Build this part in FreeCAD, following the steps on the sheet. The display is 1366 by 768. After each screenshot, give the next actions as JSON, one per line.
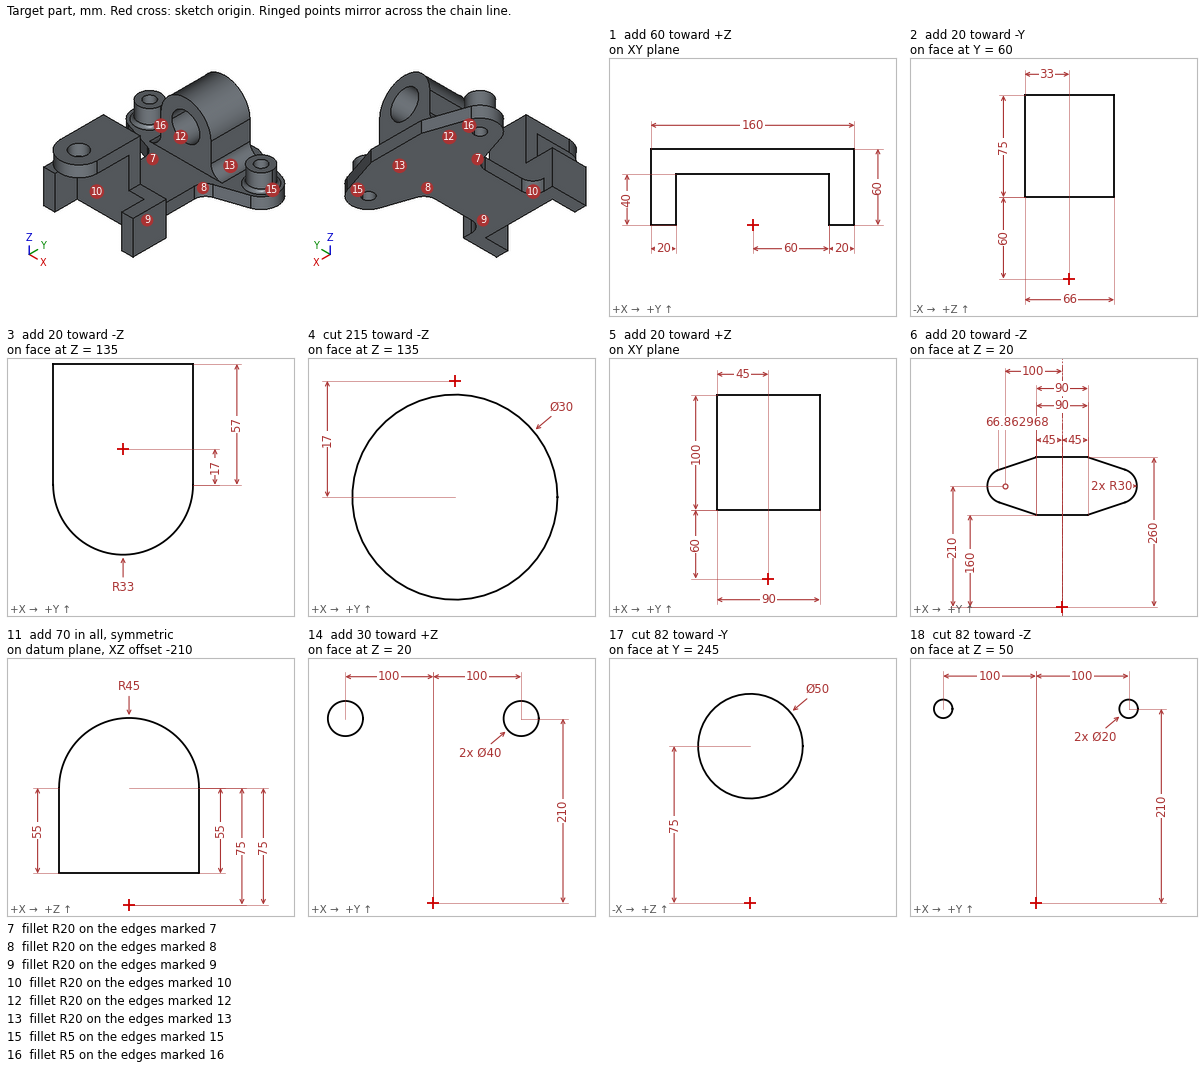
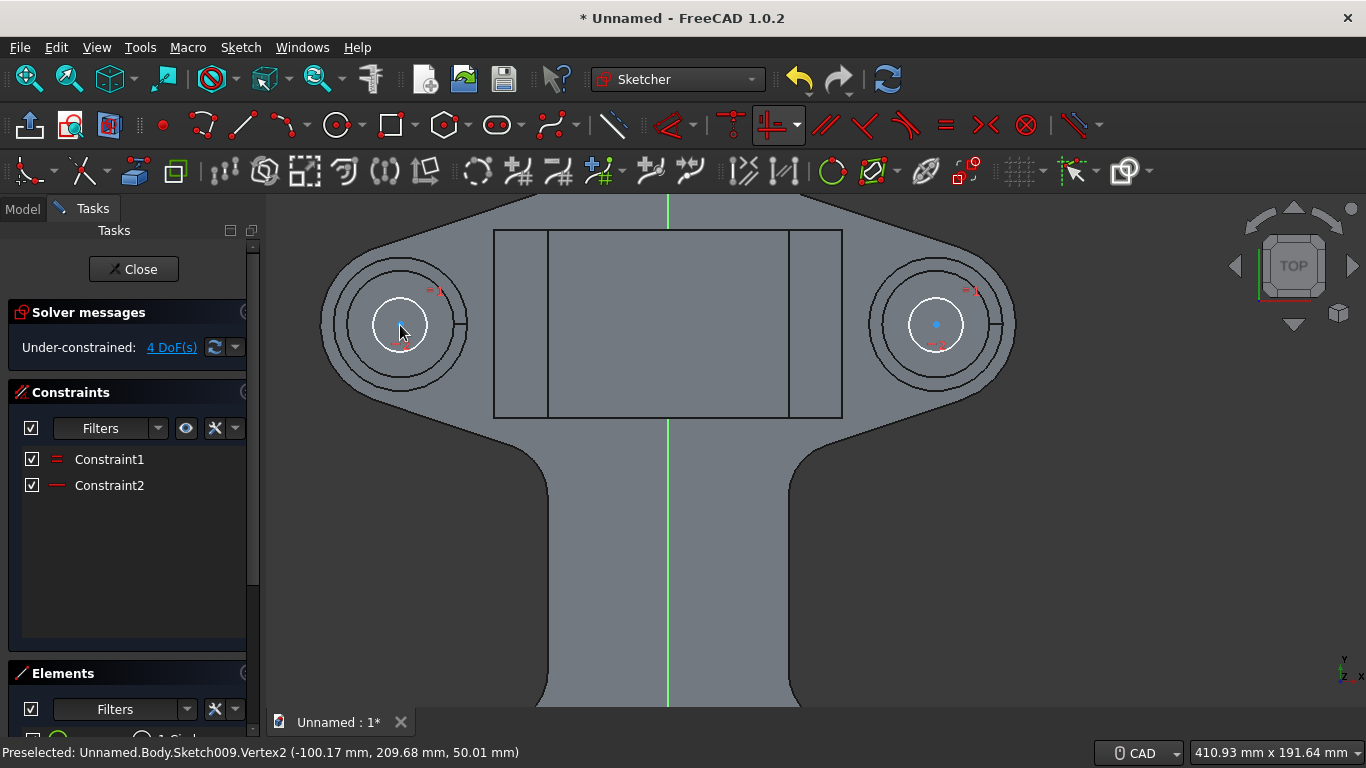
{"action": "left_click", "coordinate": [668, 126]}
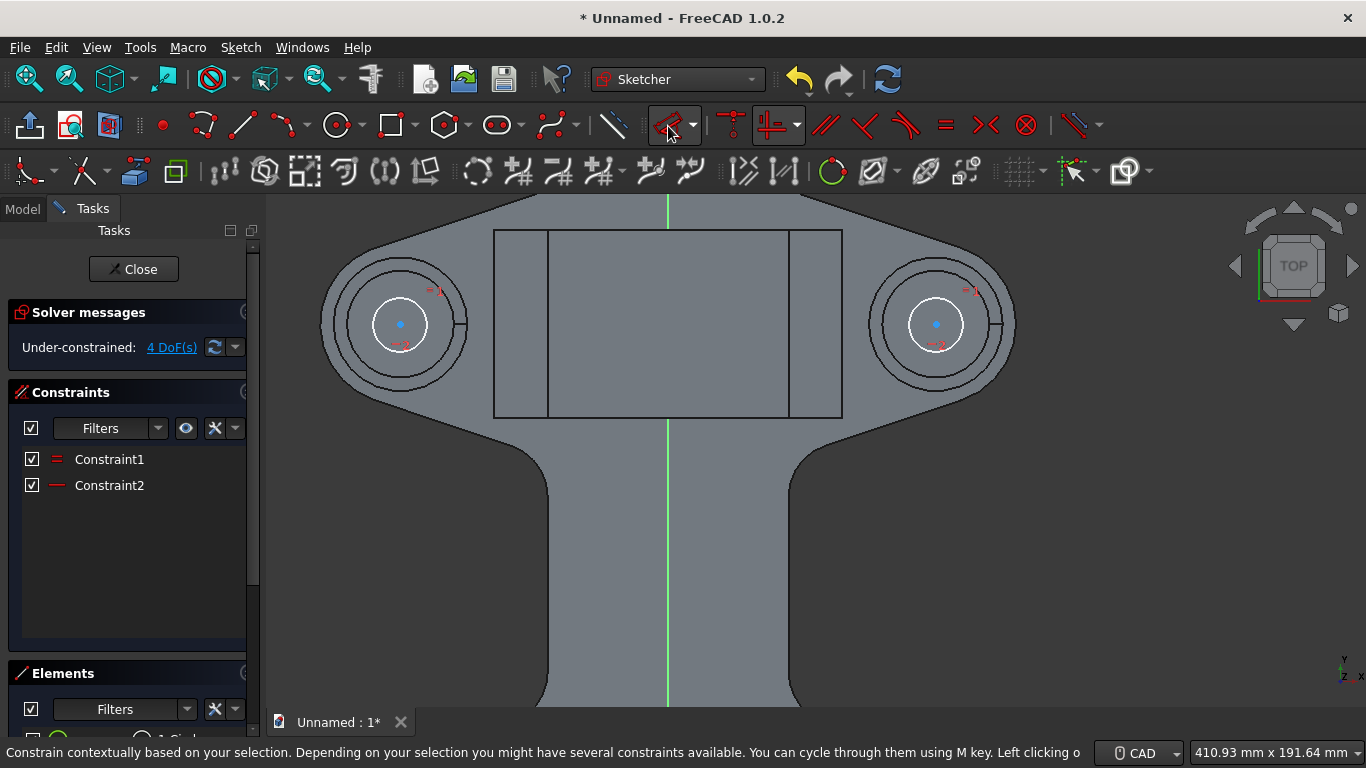
{"action": "left_click", "coordinate": [955, 306]}
{"action": "left_click", "coordinate": [978, 283]}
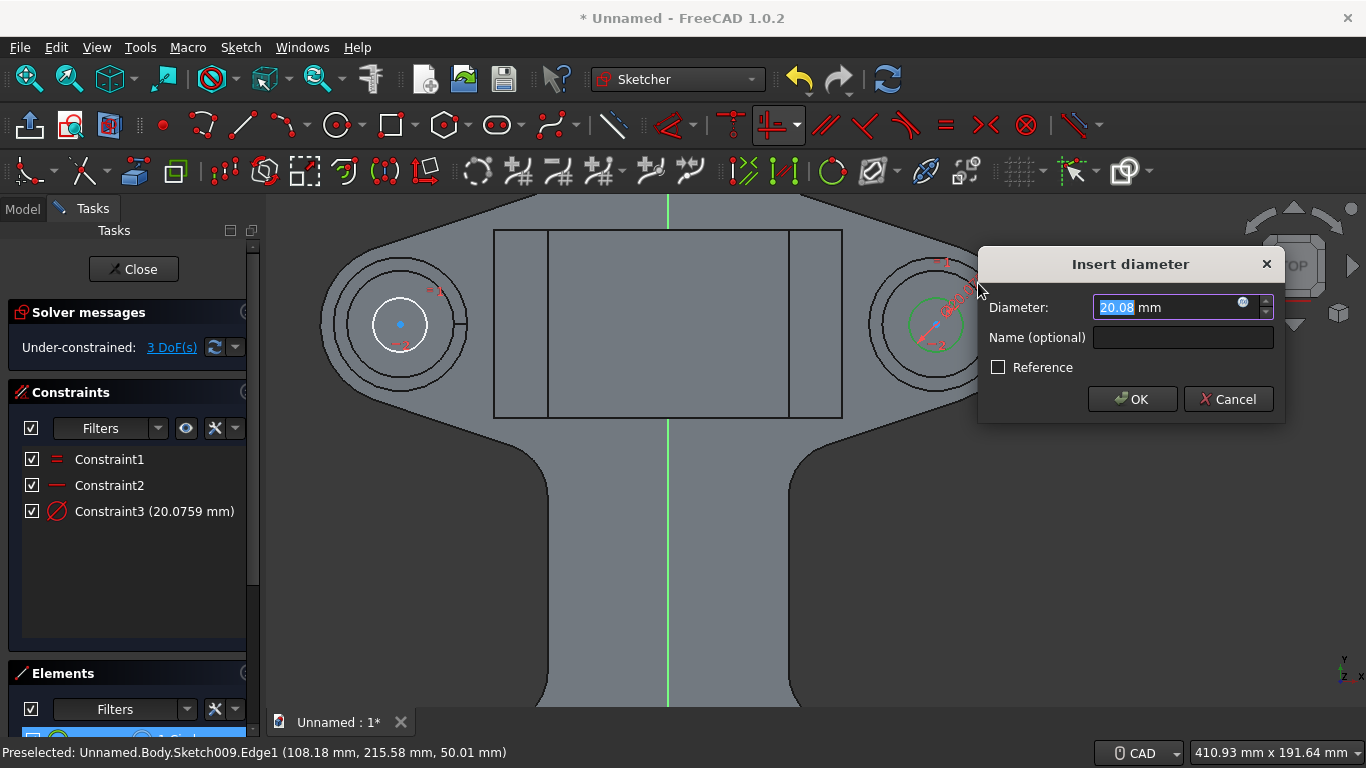
{"action": "type", "text": "20"}
{"action": "key", "text": "Return"}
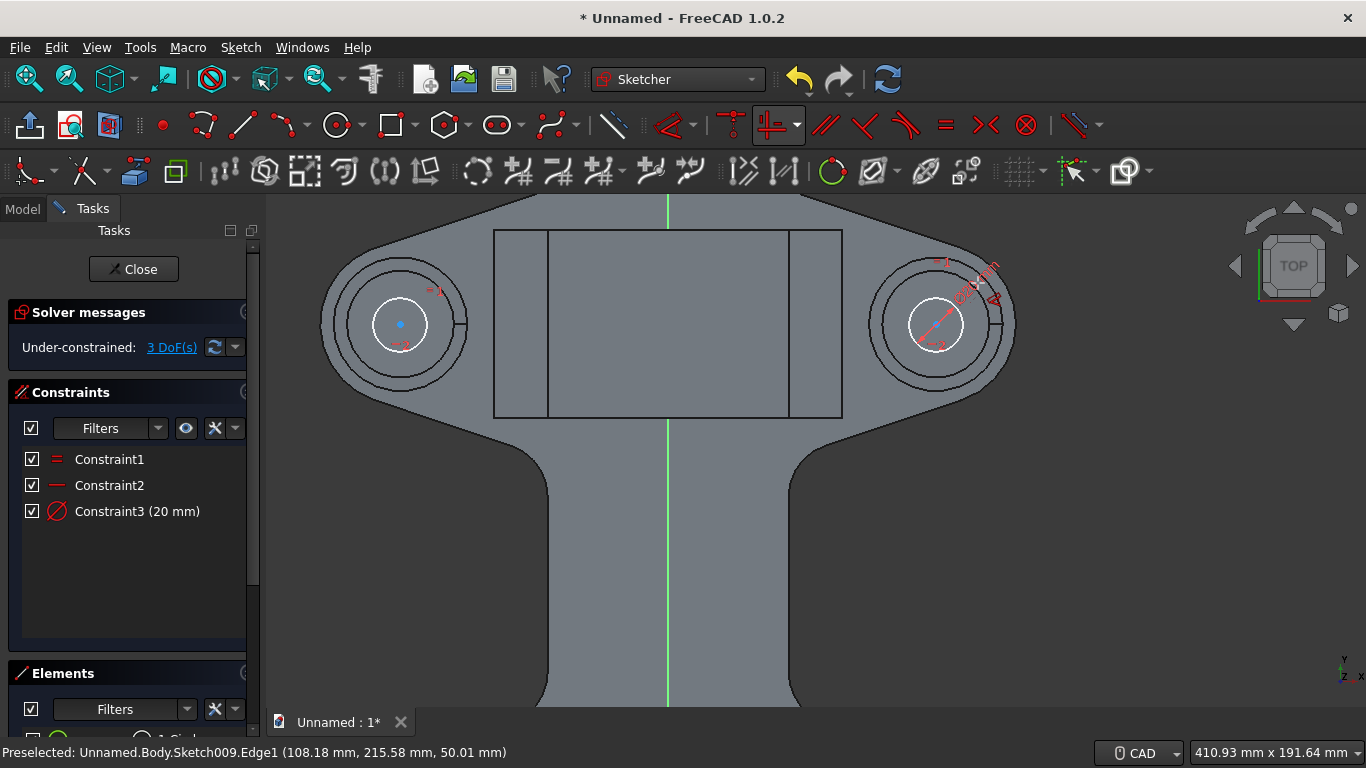
{"action": "left_click", "coordinate": [936, 325]}
{"action": "left_click", "coordinate": [802, 291]}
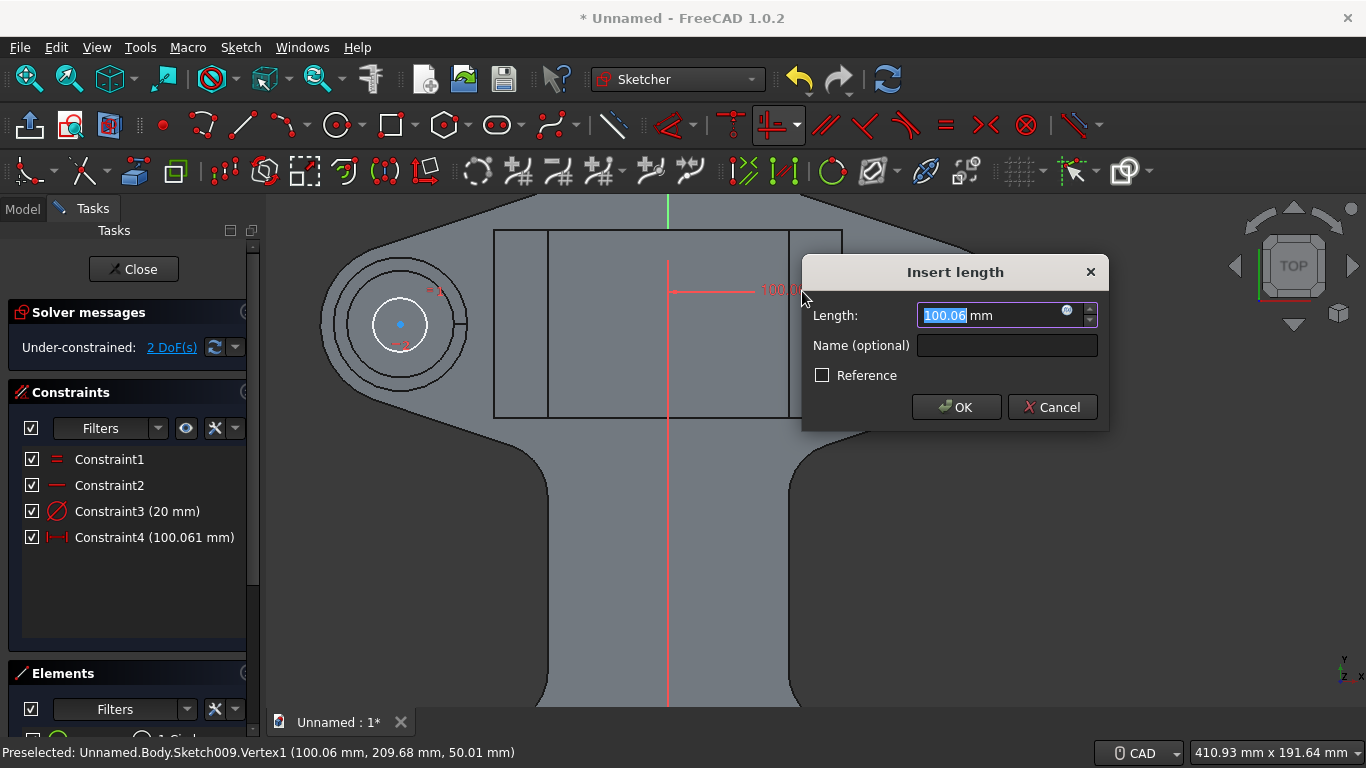
{"action": "type", "text": "100"}
{"action": "key", "text": "Return"}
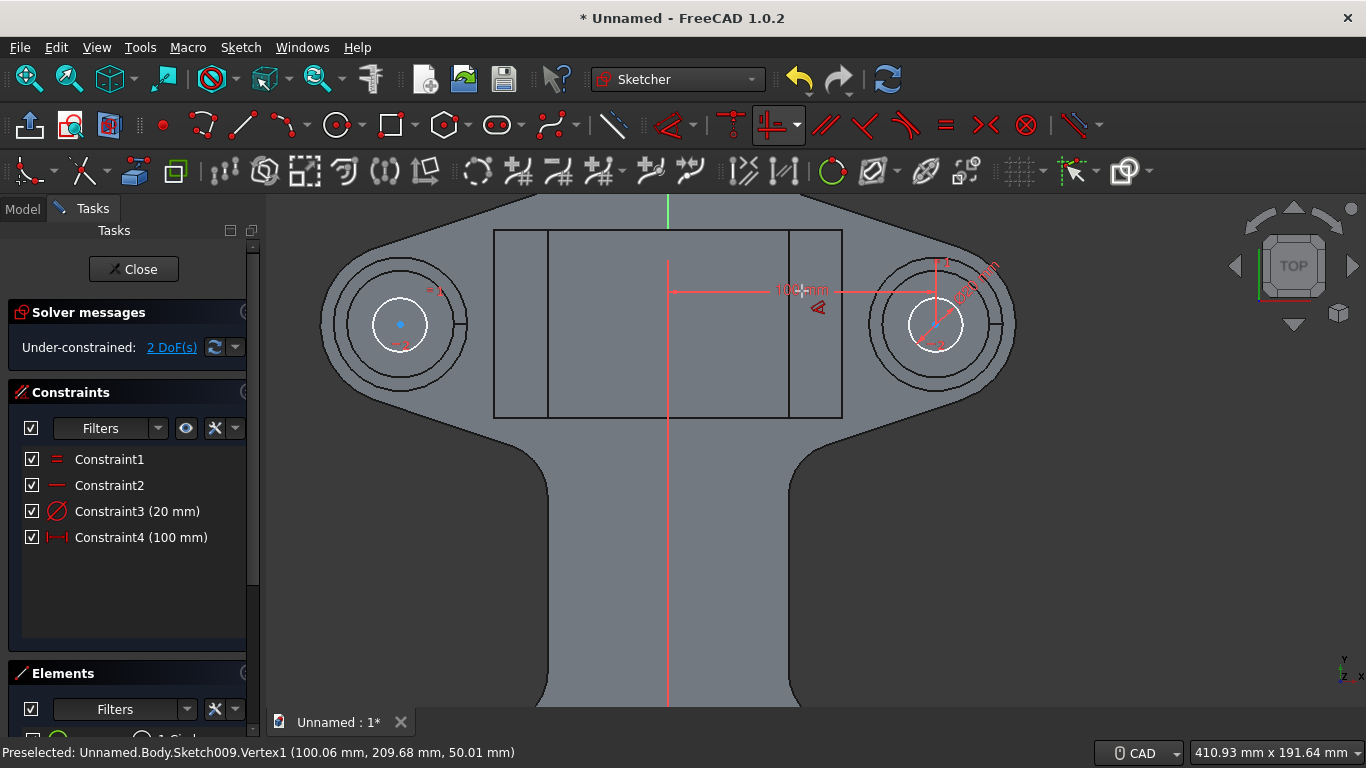
{"action": "left_click", "coordinate": [936, 325]}
{"action": "left_click", "coordinate": [970, 502]}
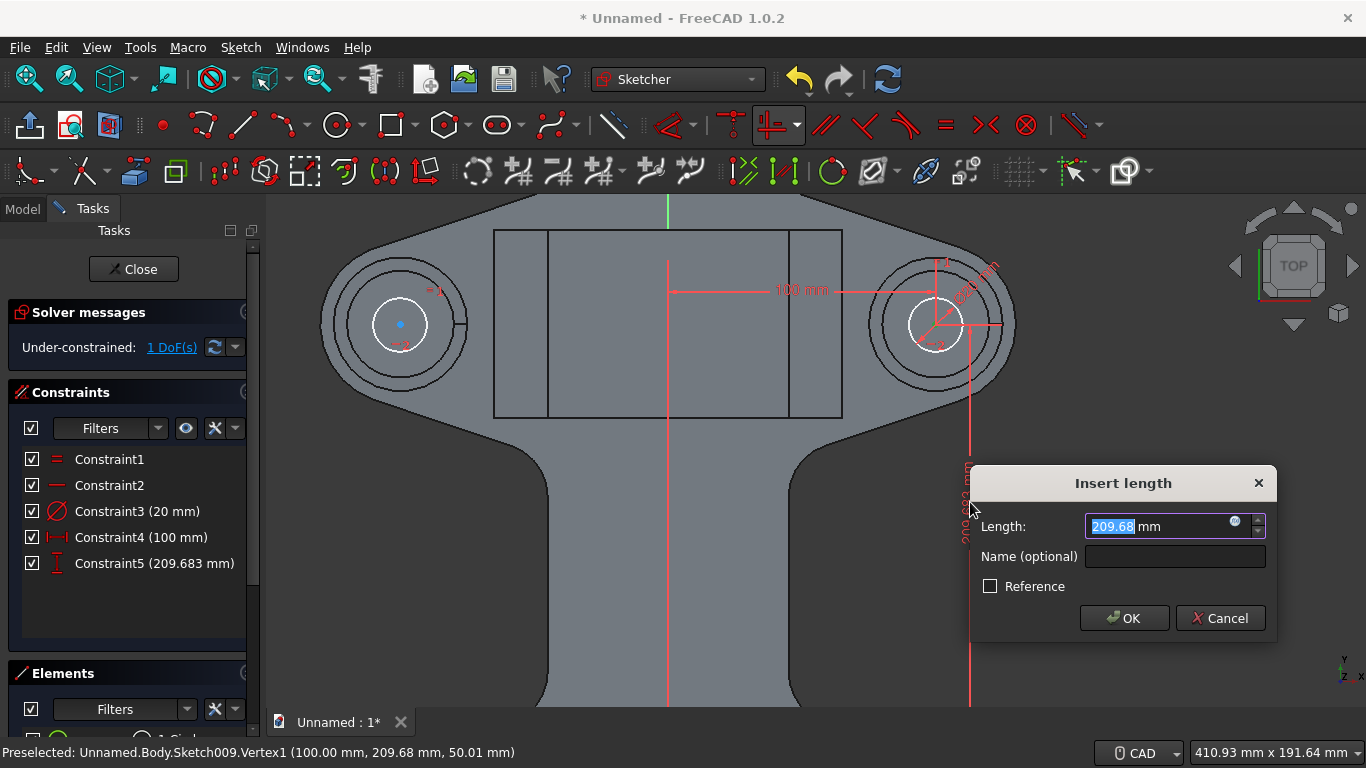
{"action": "type", "text": "210"}
{"action": "key", "text": "Return"}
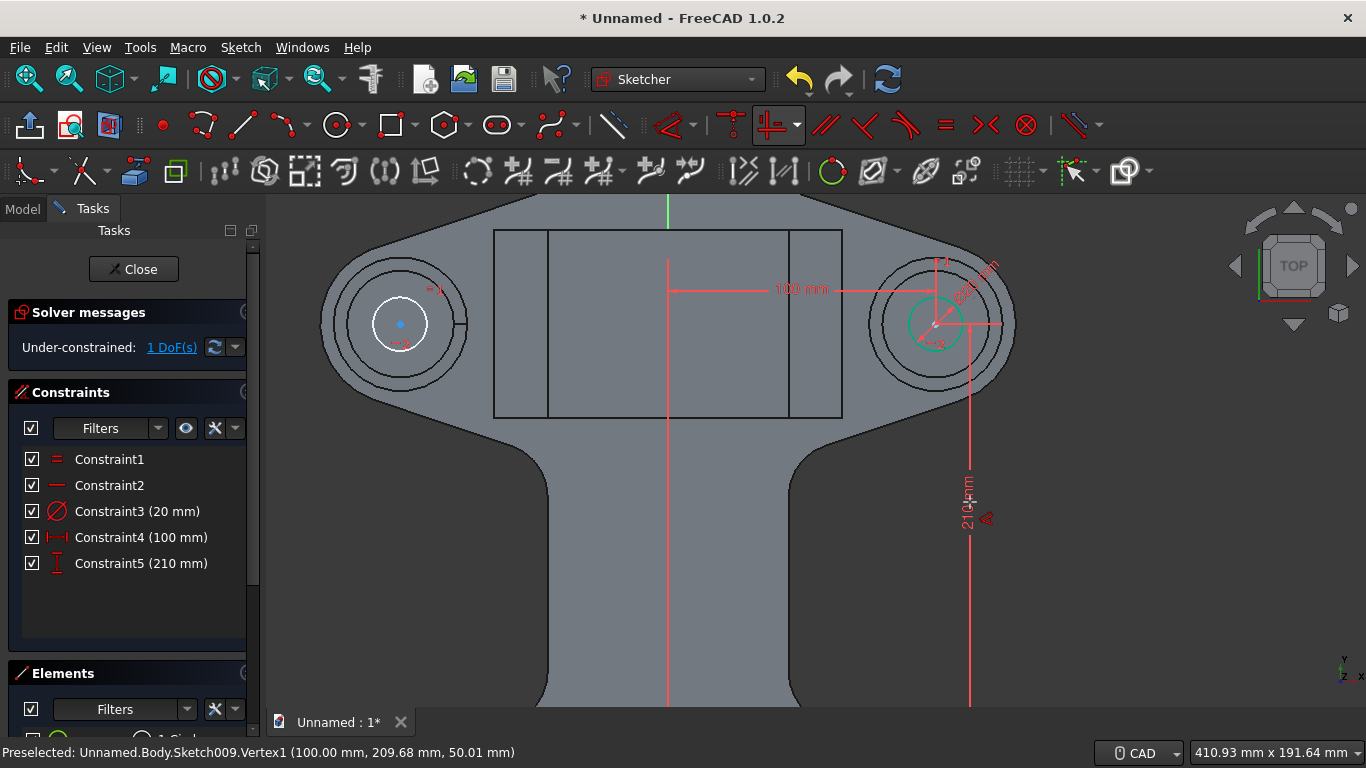
{"action": "left_click", "coordinate": [400, 324]}
{"action": "left_click", "coordinate": [534, 290]}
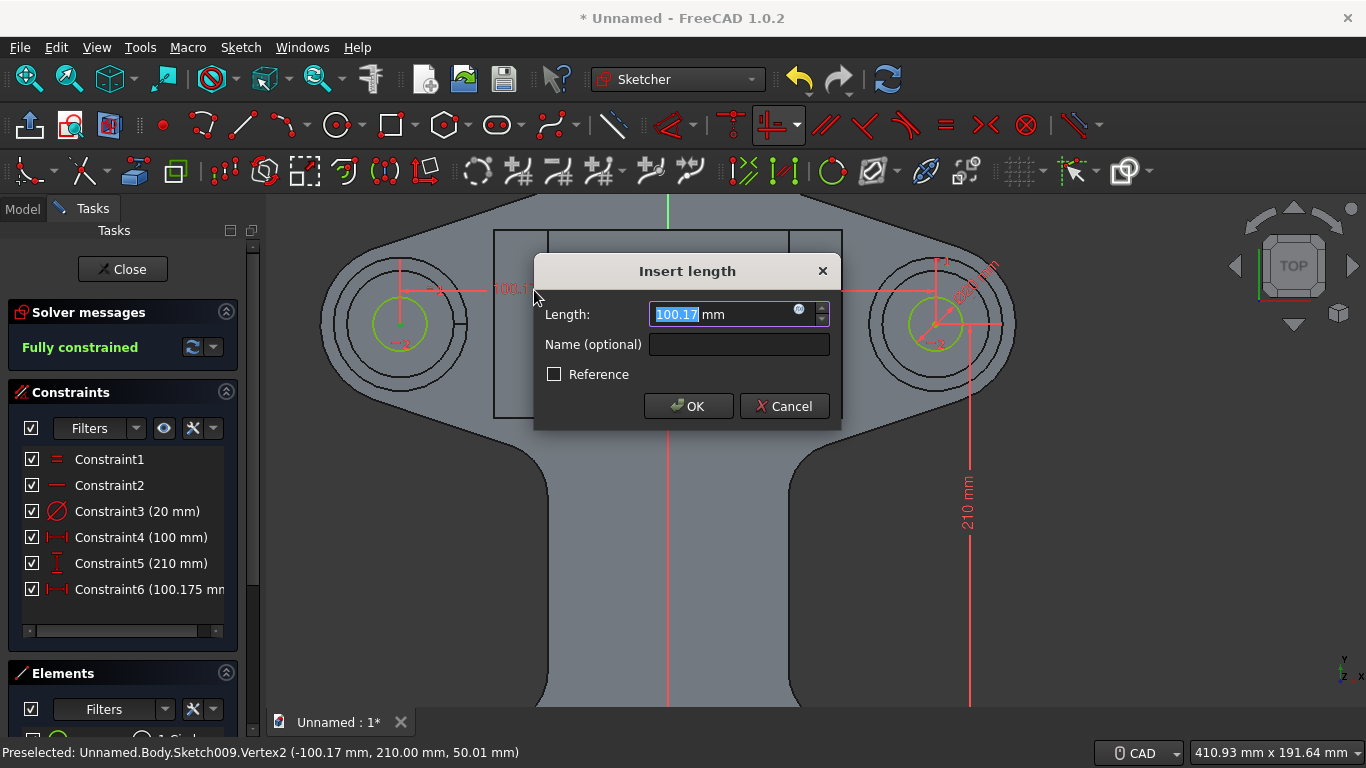
{"action": "type", "text": "100"}
{"action": "key", "text": "Return"}
{"action": "key", "text": "Escape"}